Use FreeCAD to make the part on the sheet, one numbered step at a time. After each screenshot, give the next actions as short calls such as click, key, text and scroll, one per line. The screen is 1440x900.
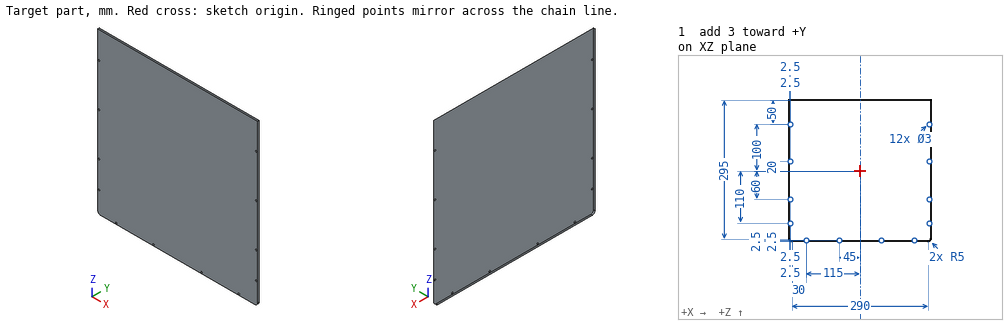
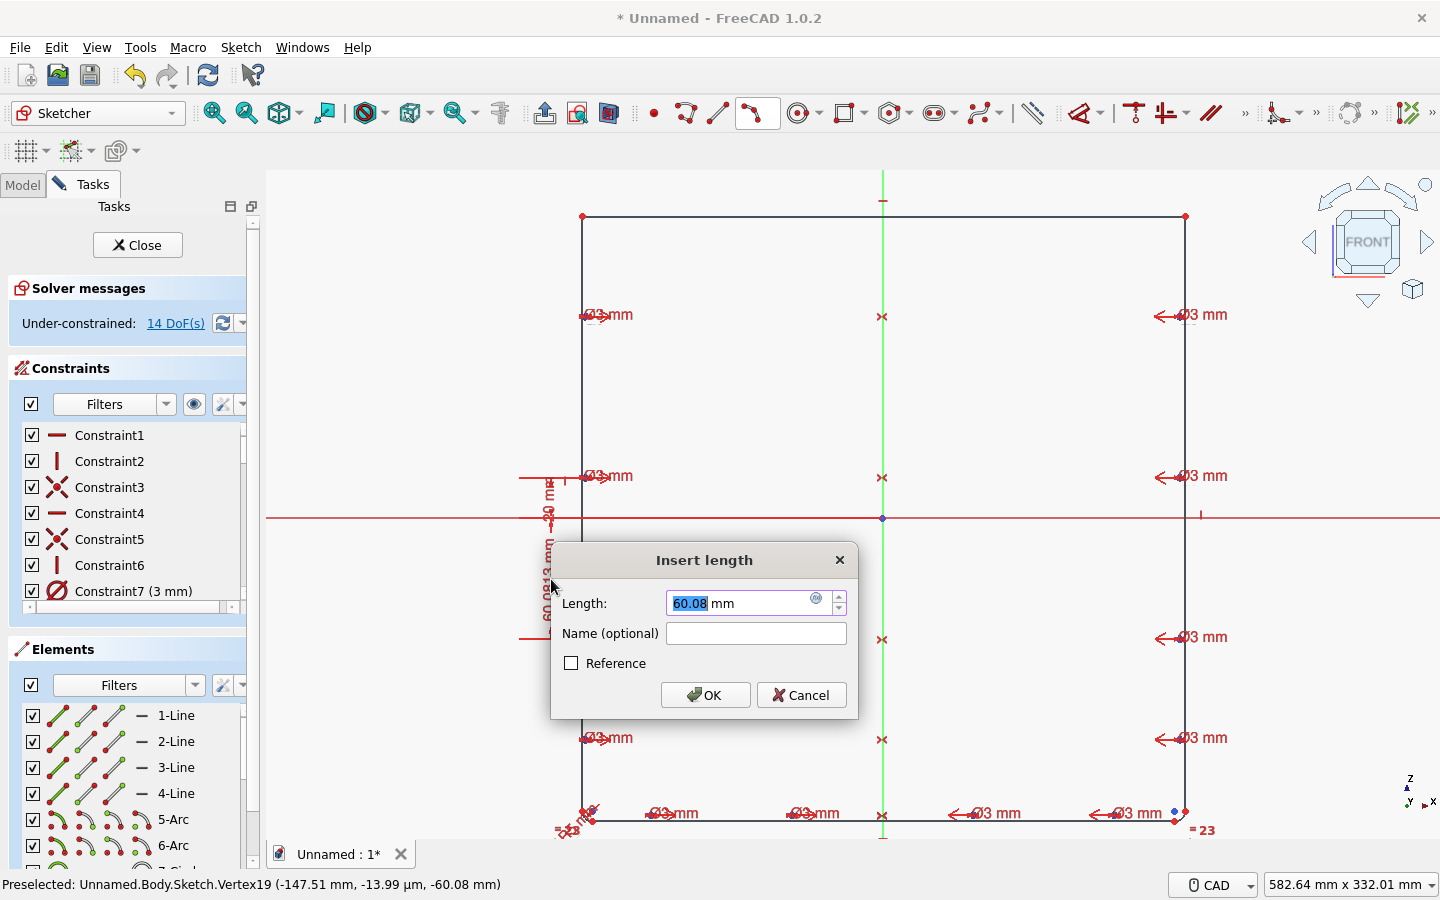
text(60)
key(Return)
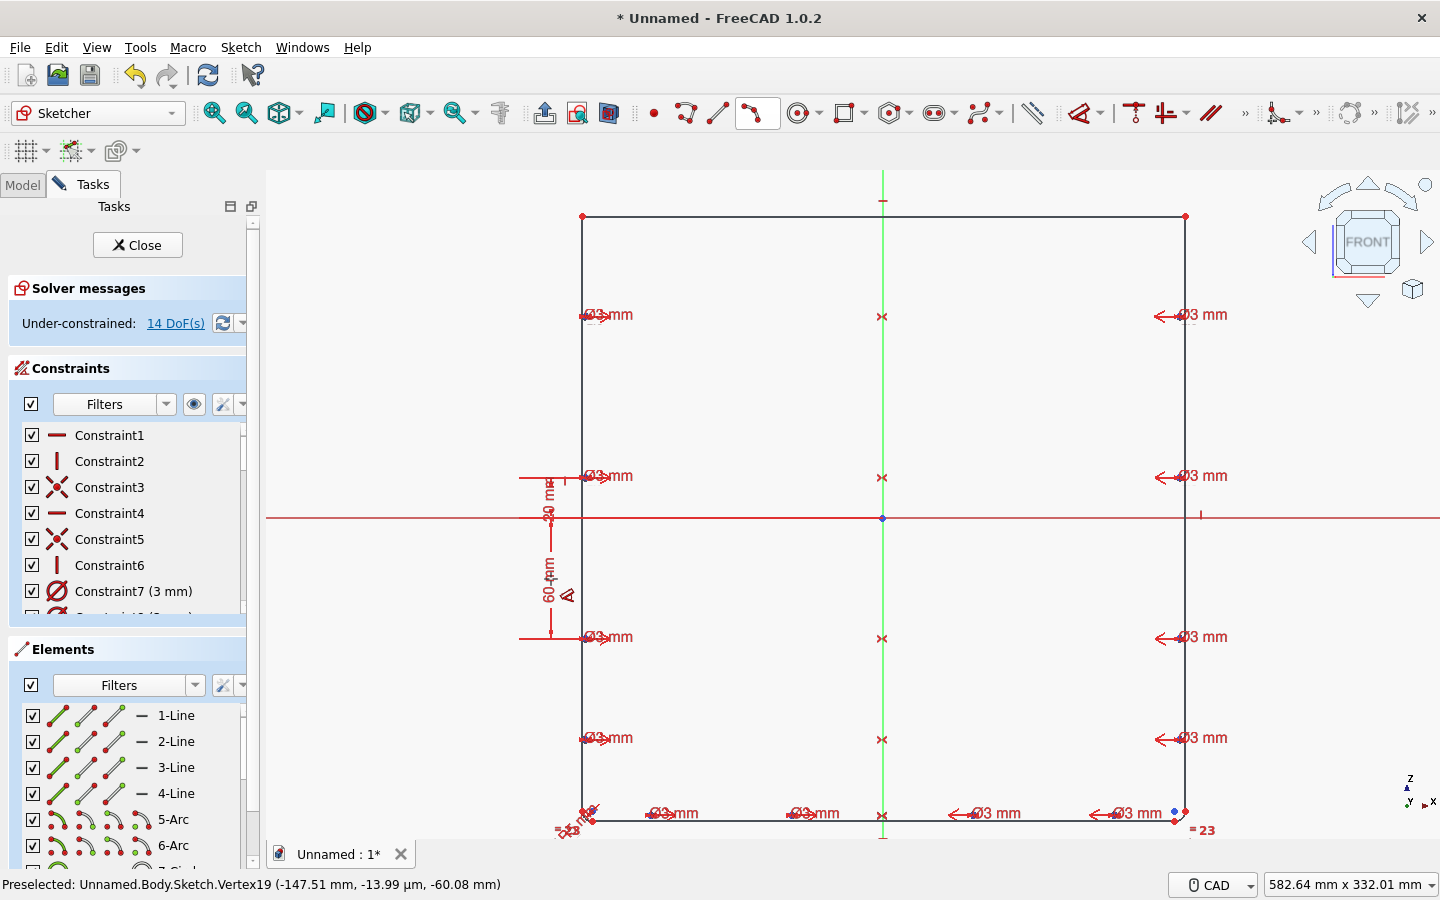
scroll(585, 477, down, 2)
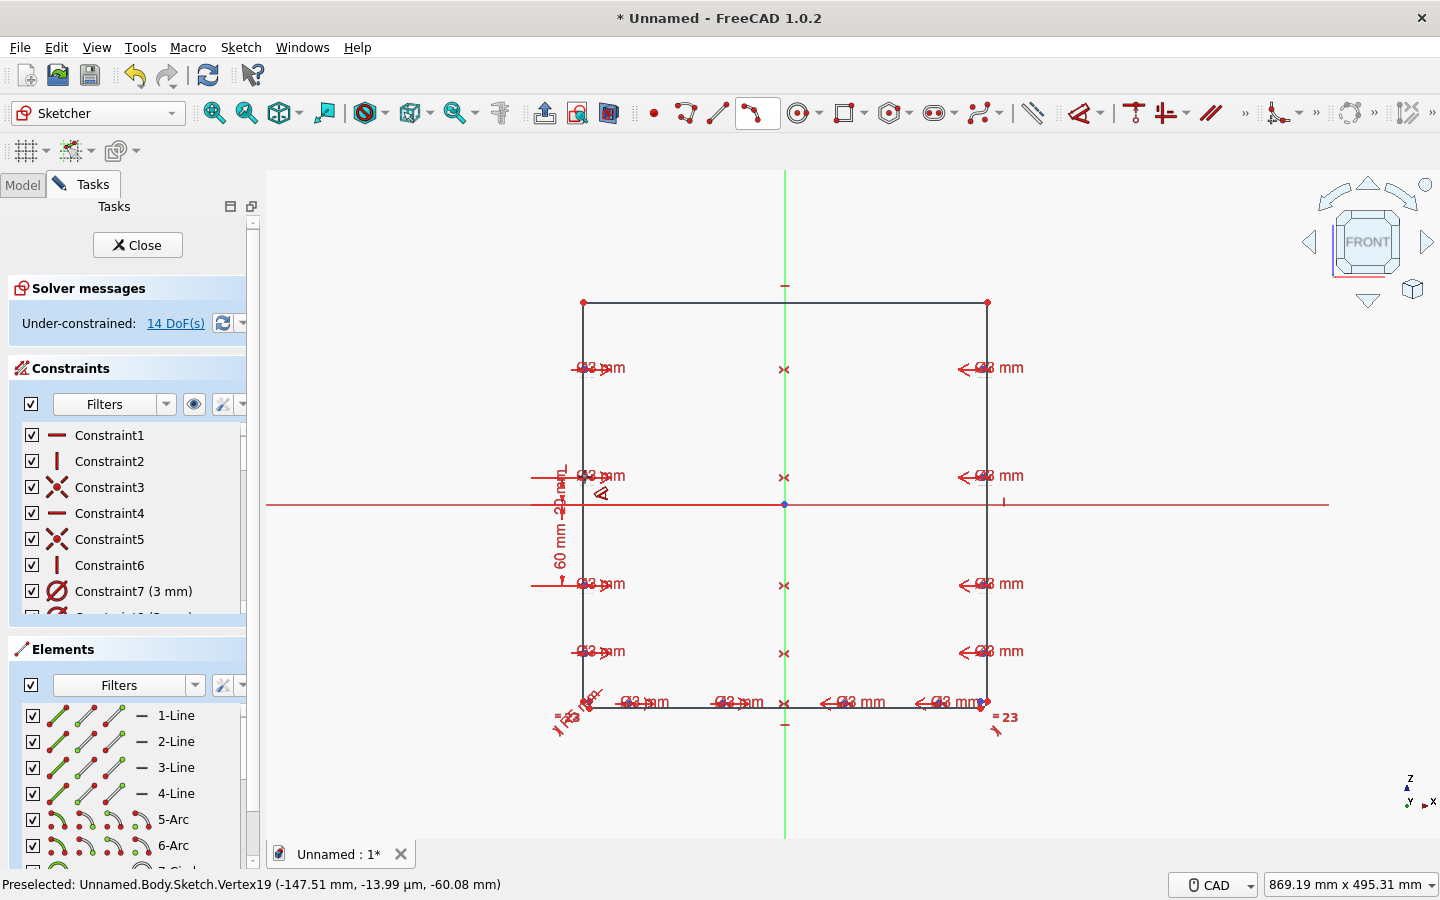
click(724, 704)
click(754, 738)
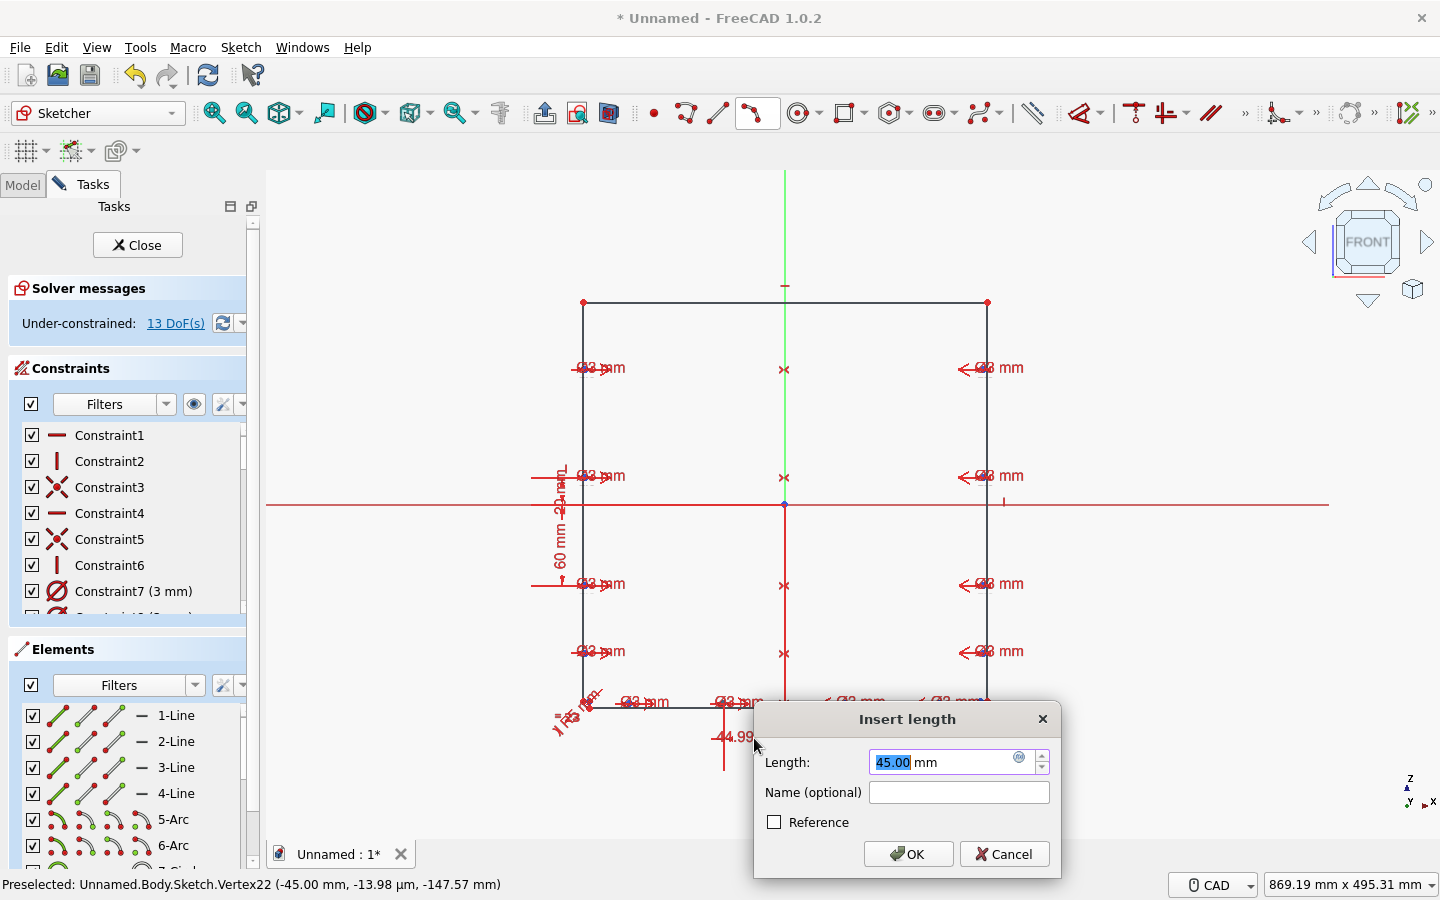
text(45)
key(Return)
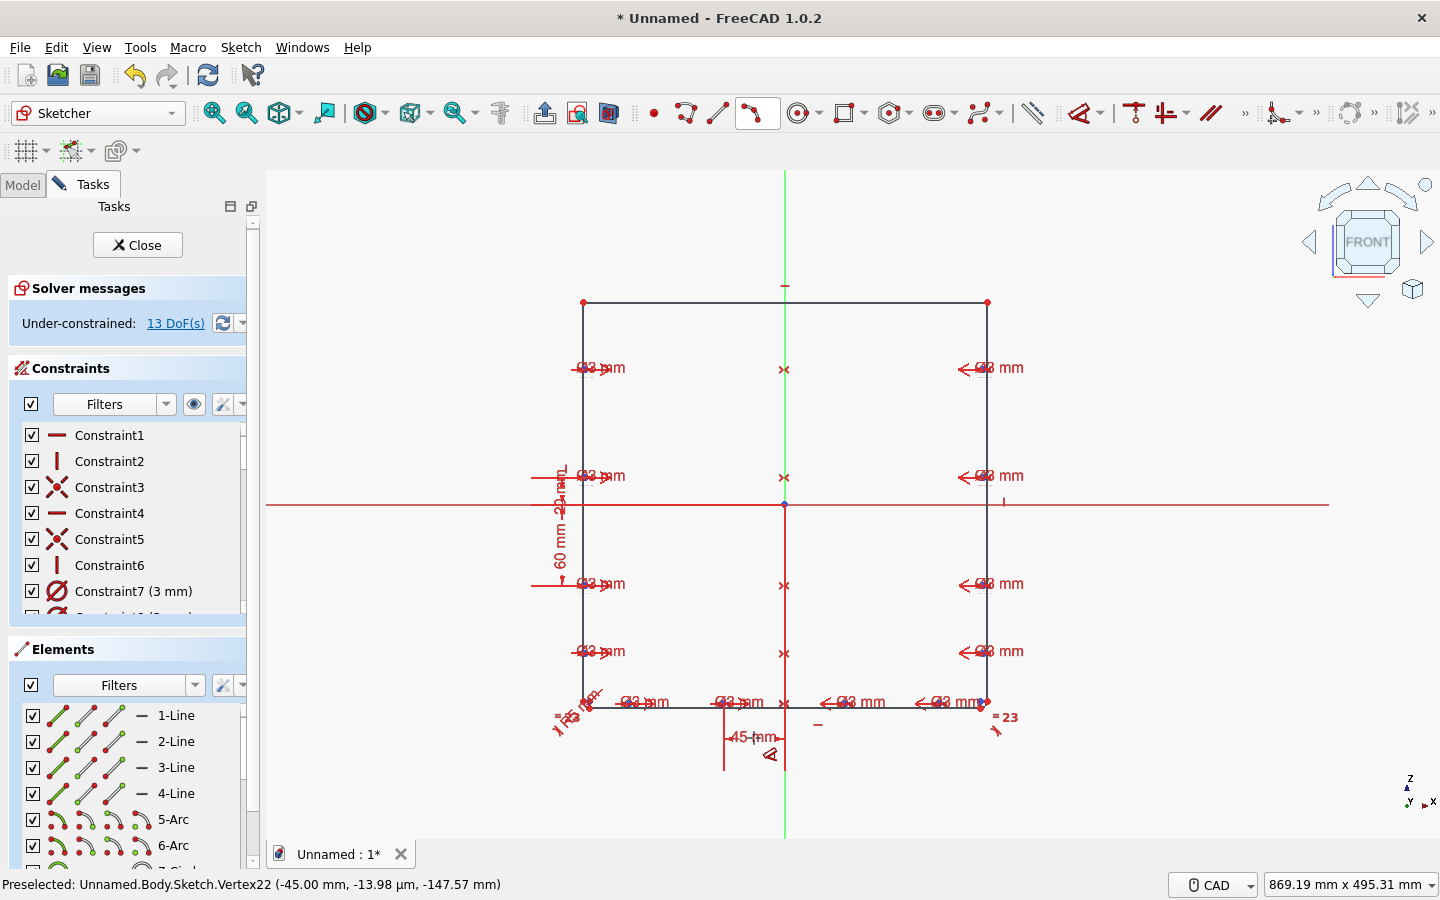
click(863, 708)
click(875, 742)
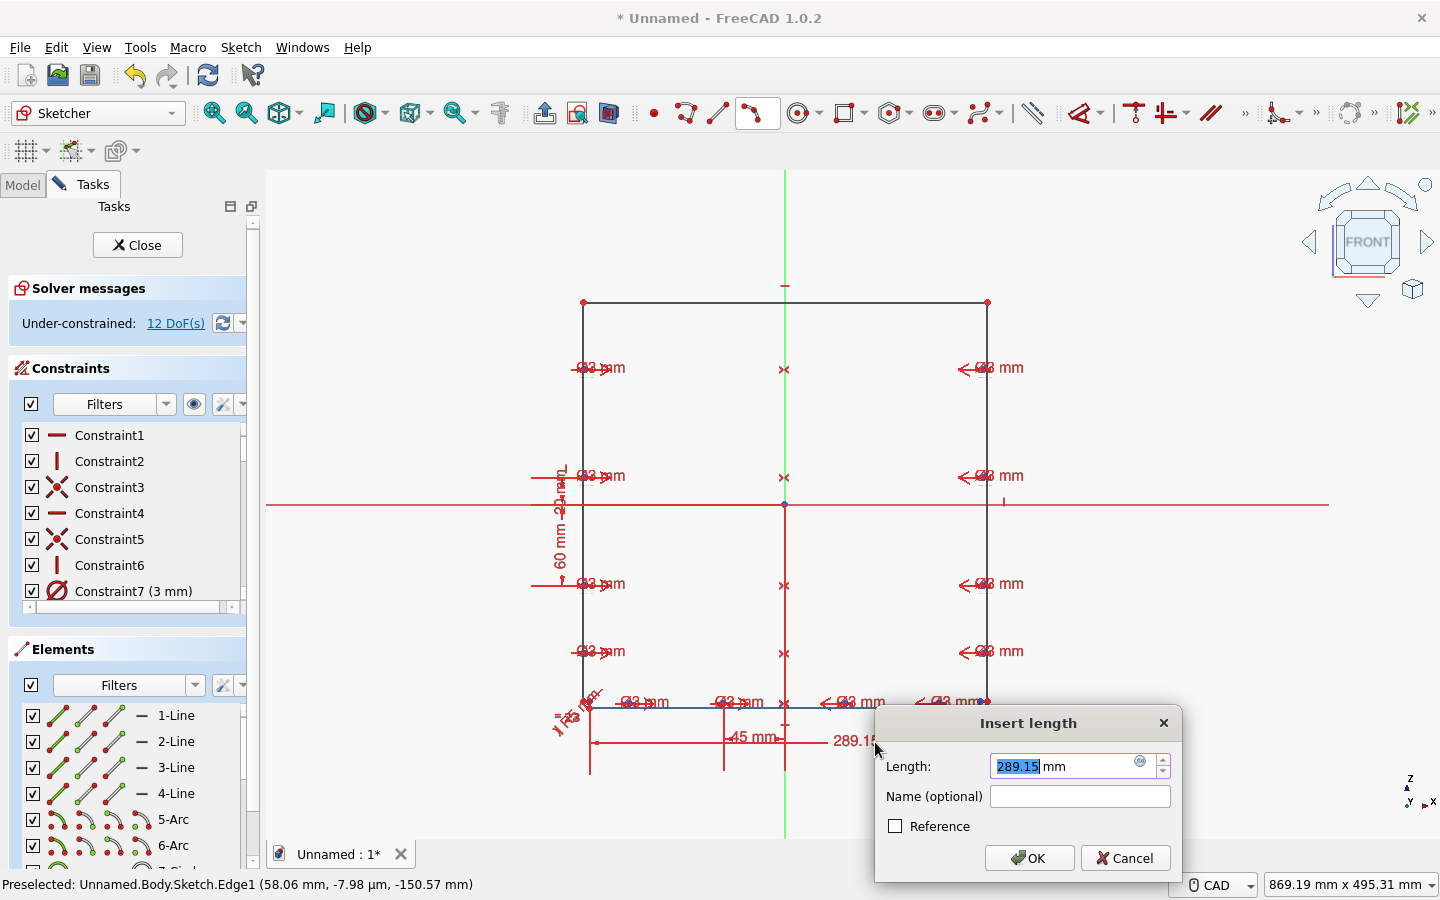
text(290)
key(Return)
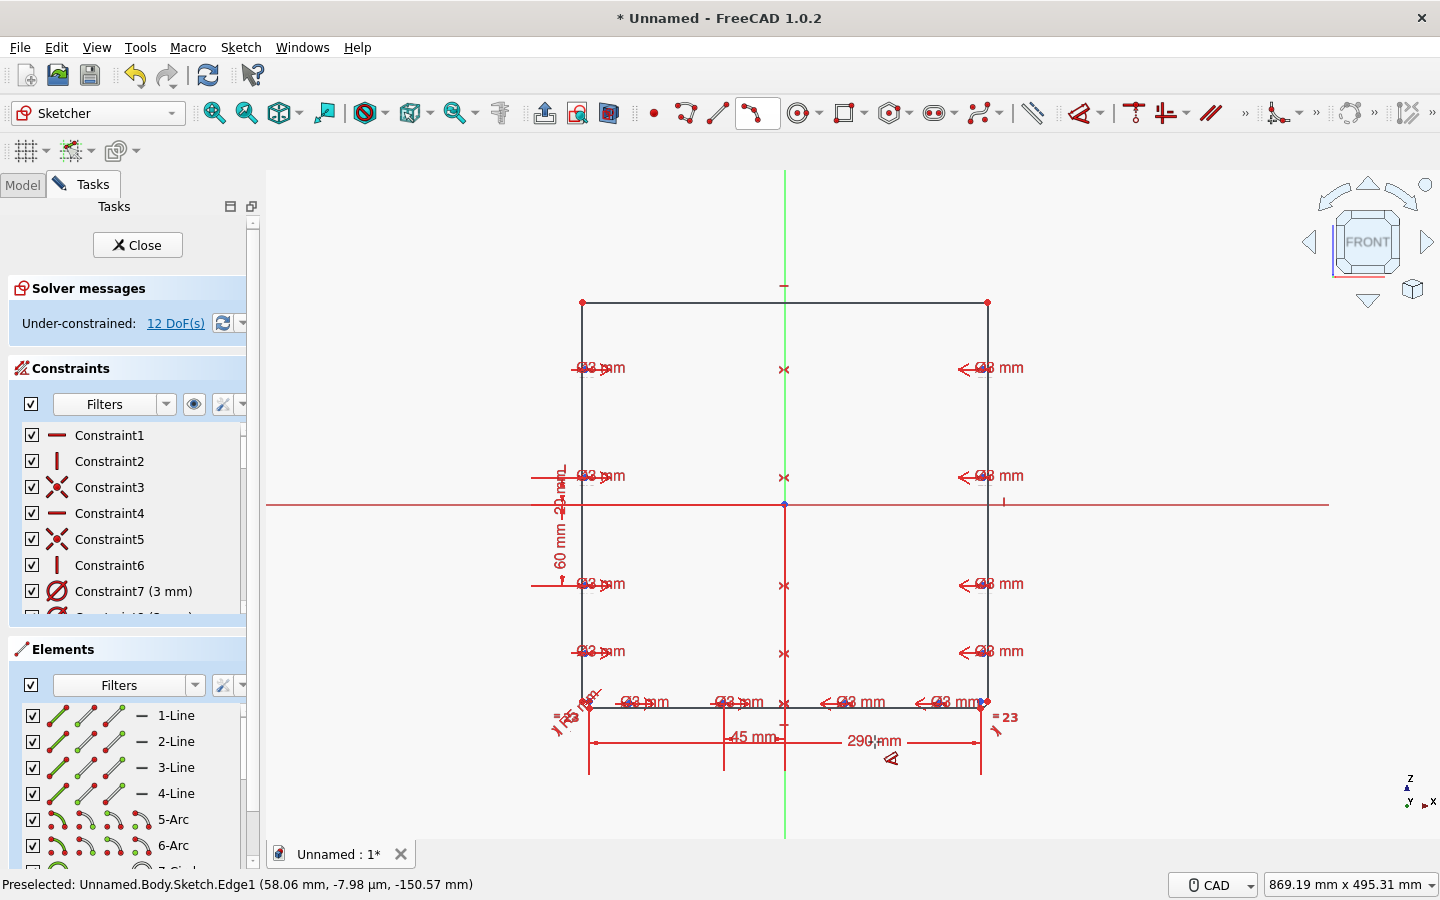
click(582, 422)
click(548, 410)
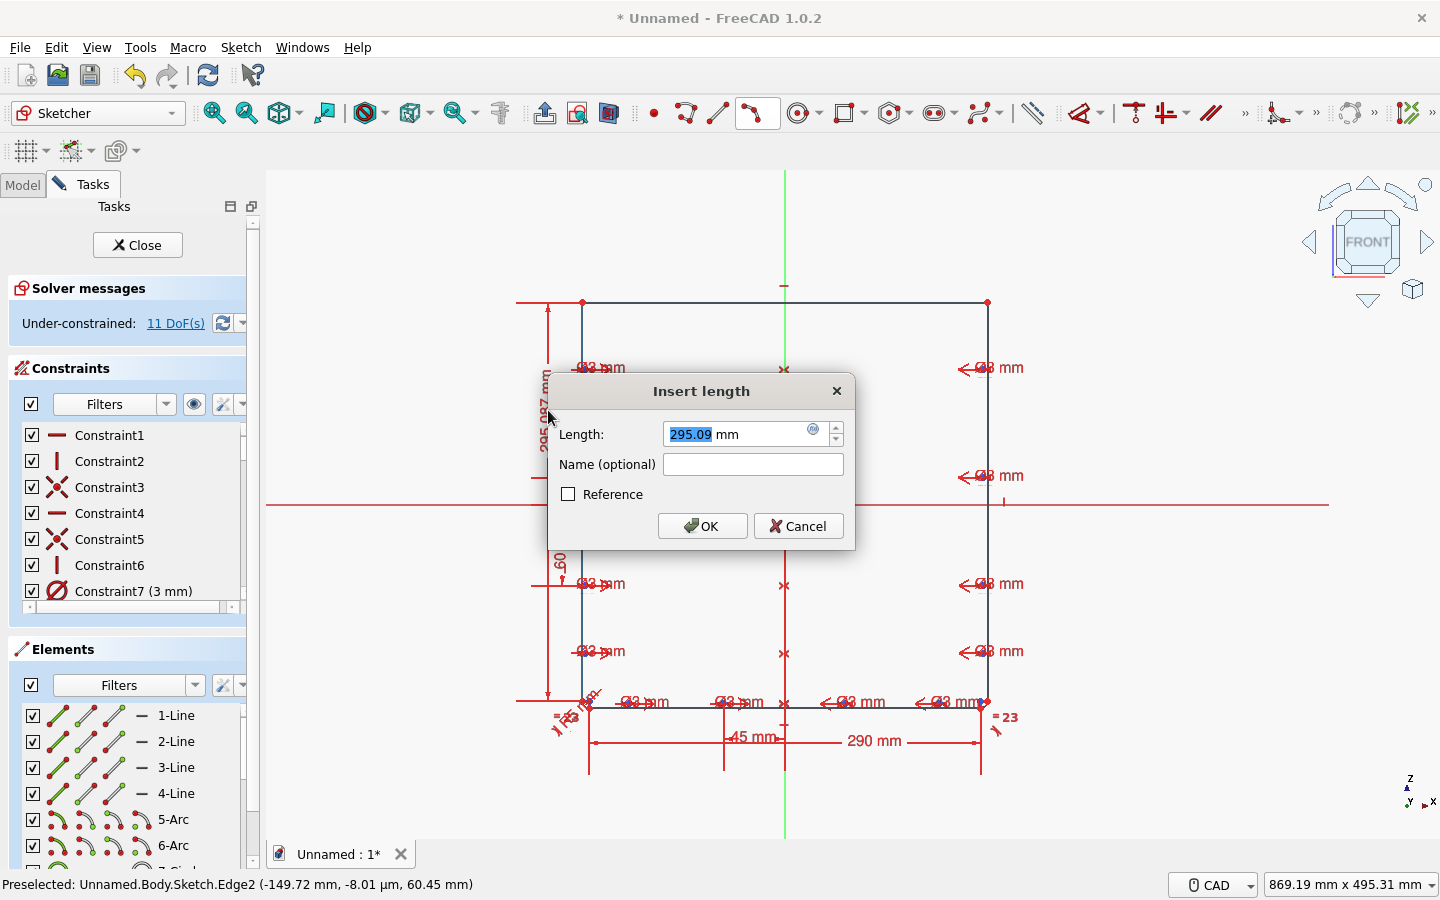
text(295)
key(Return)